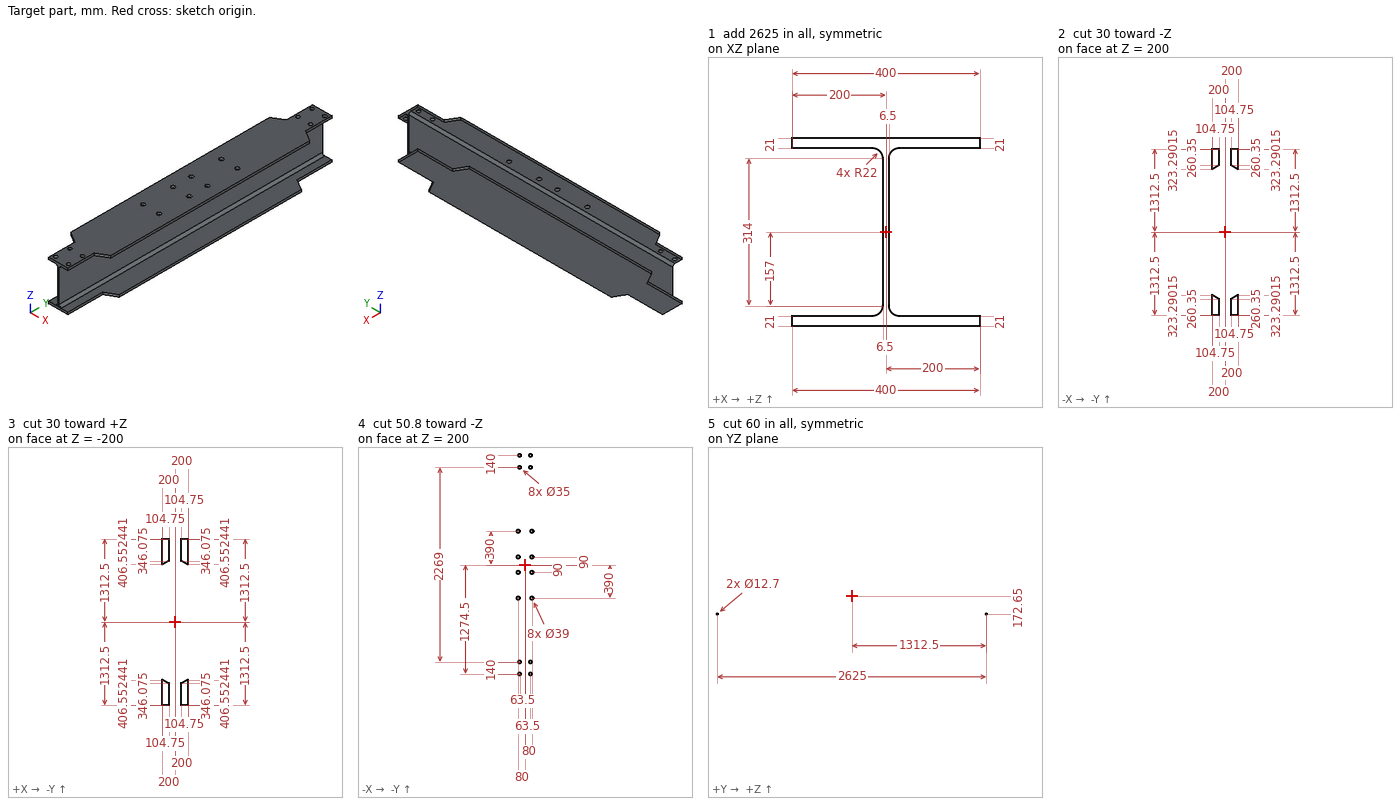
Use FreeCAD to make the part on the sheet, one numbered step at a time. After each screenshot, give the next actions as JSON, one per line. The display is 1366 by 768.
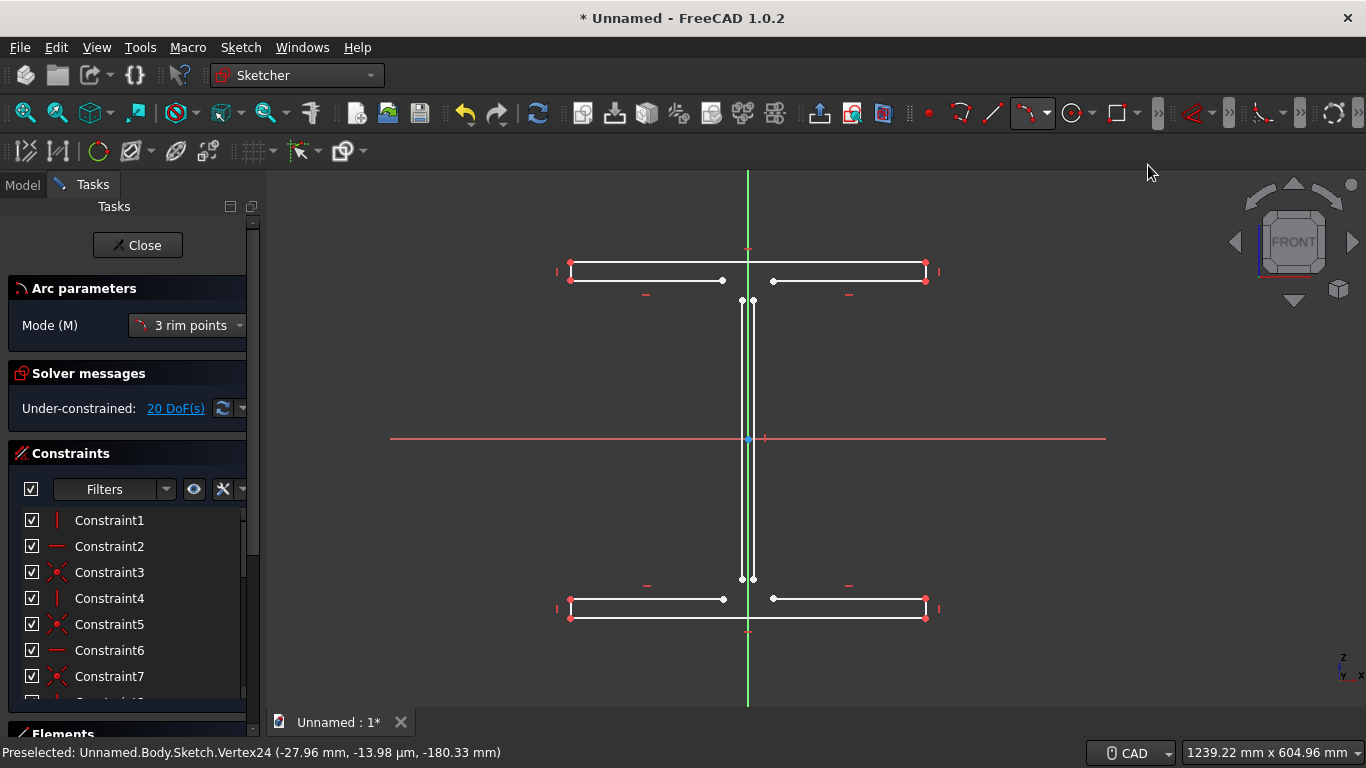
{"action": "scroll", "coordinate": [742, 300], "scroll_direction": "up", "scroll_amount": 6}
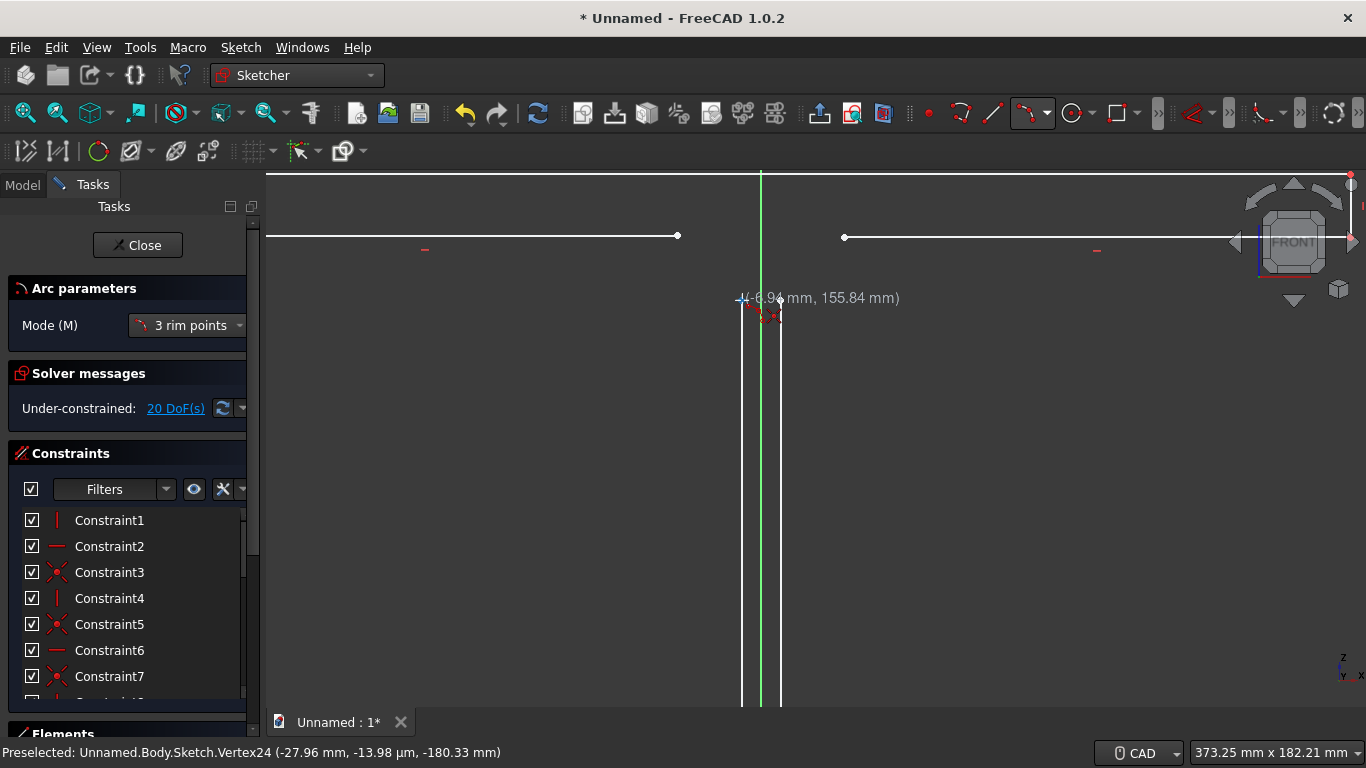
{"action": "left_click", "coordinate": [742, 300]}
{"action": "left_click", "coordinate": [677, 236]}
{"action": "left_click", "coordinate": [723, 253]}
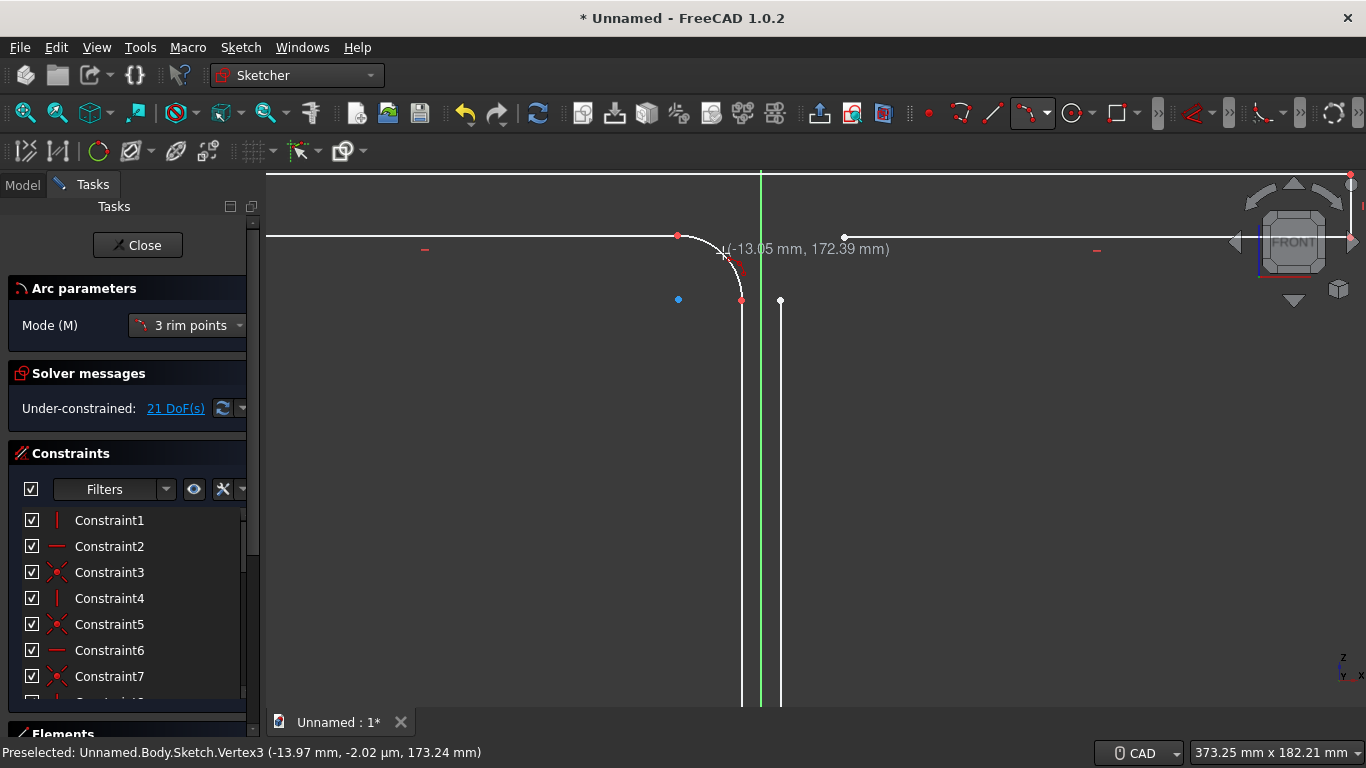
{"action": "left_click", "coordinate": [844, 237]}
{"action": "left_click", "coordinate": [781, 301]}
{"action": "left_click", "coordinate": [800, 253]}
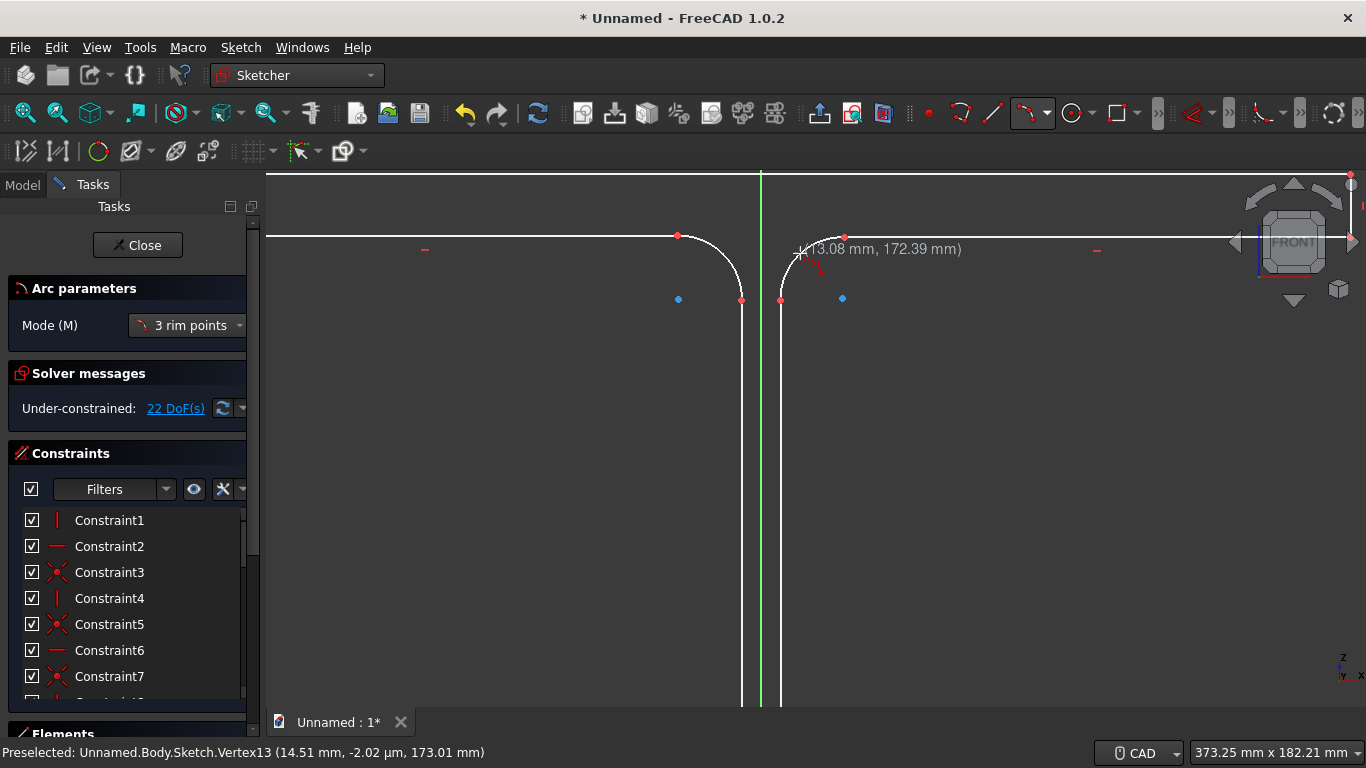
{"action": "scroll", "coordinate": [741, 299], "scroll_direction": "down", "scroll_amount": 6}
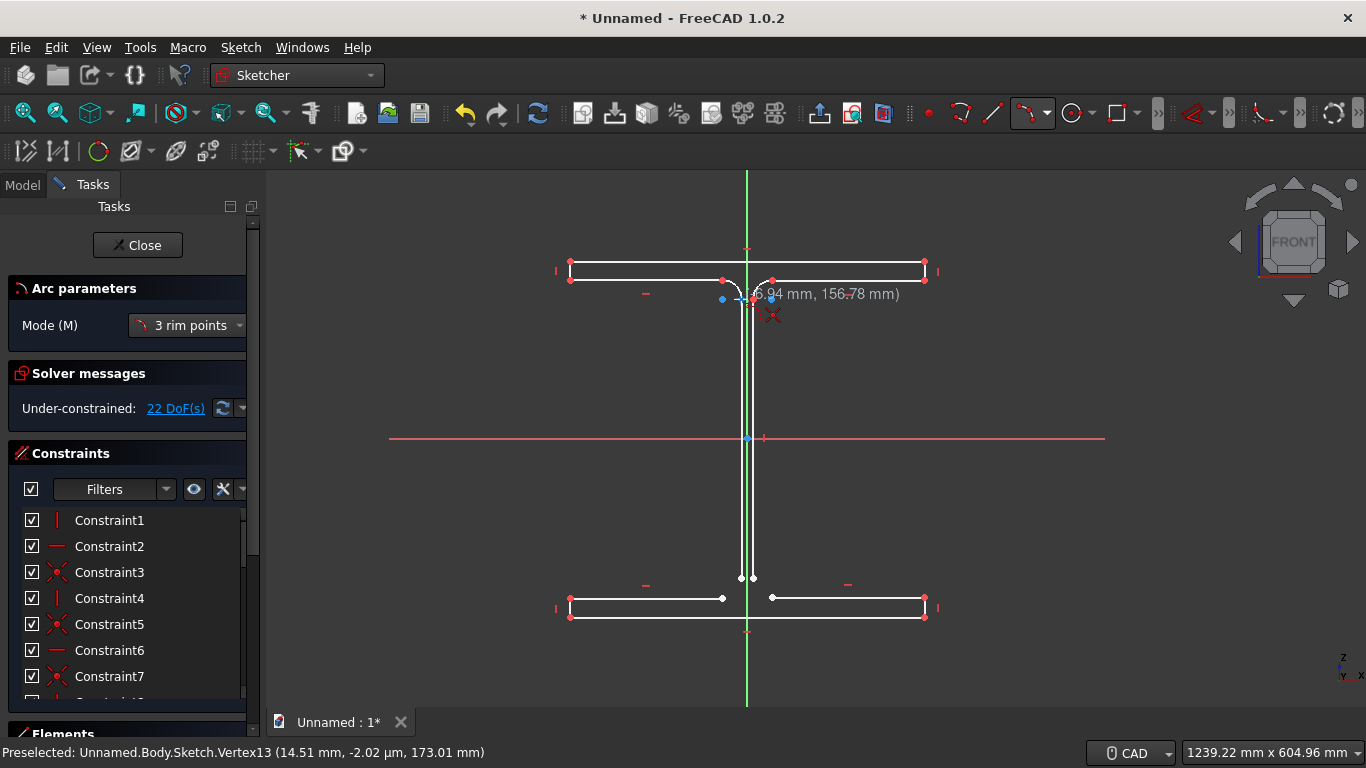
{"action": "scroll", "coordinate": [753, 578], "scroll_direction": "up", "scroll_amount": 6}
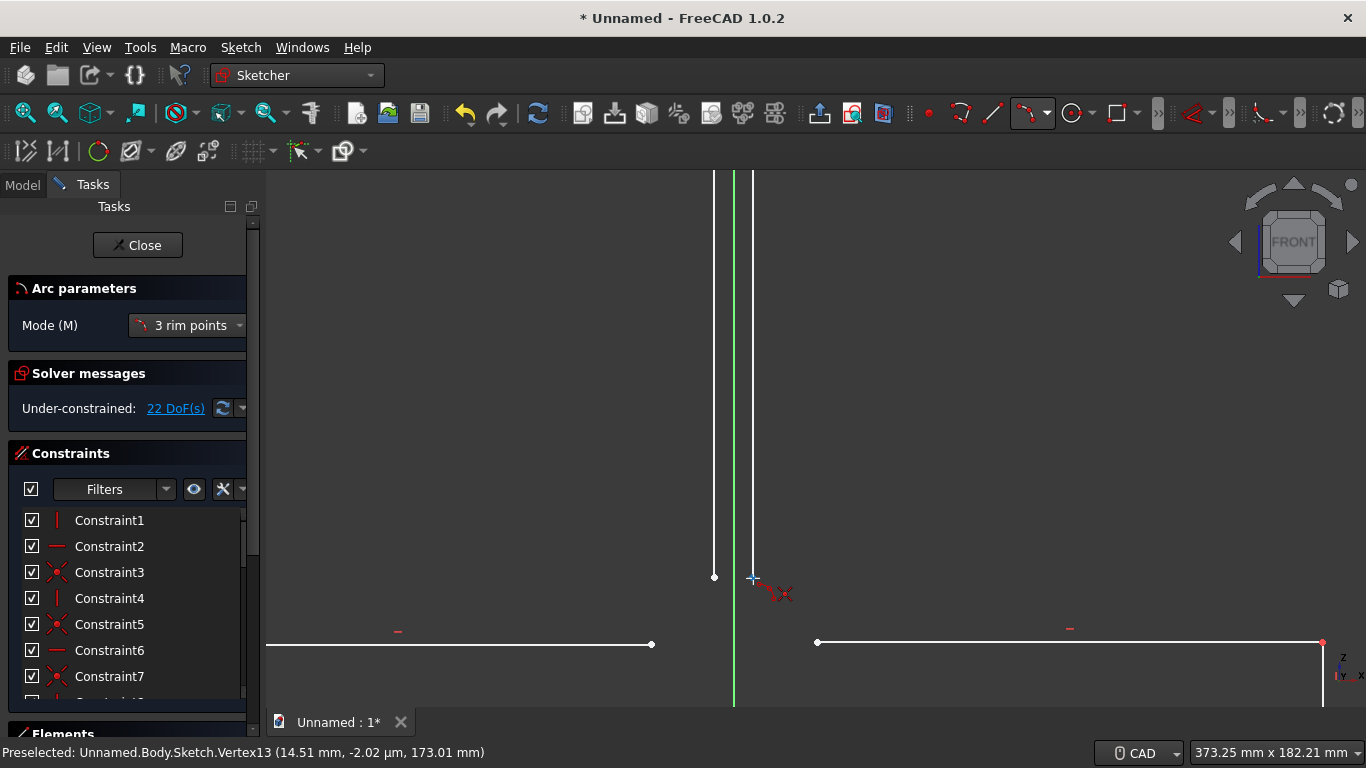
{"action": "left_click", "coordinate": [753, 578]}
{"action": "left_click", "coordinate": [818, 642]}
{"action": "left_click", "coordinate": [772, 622]}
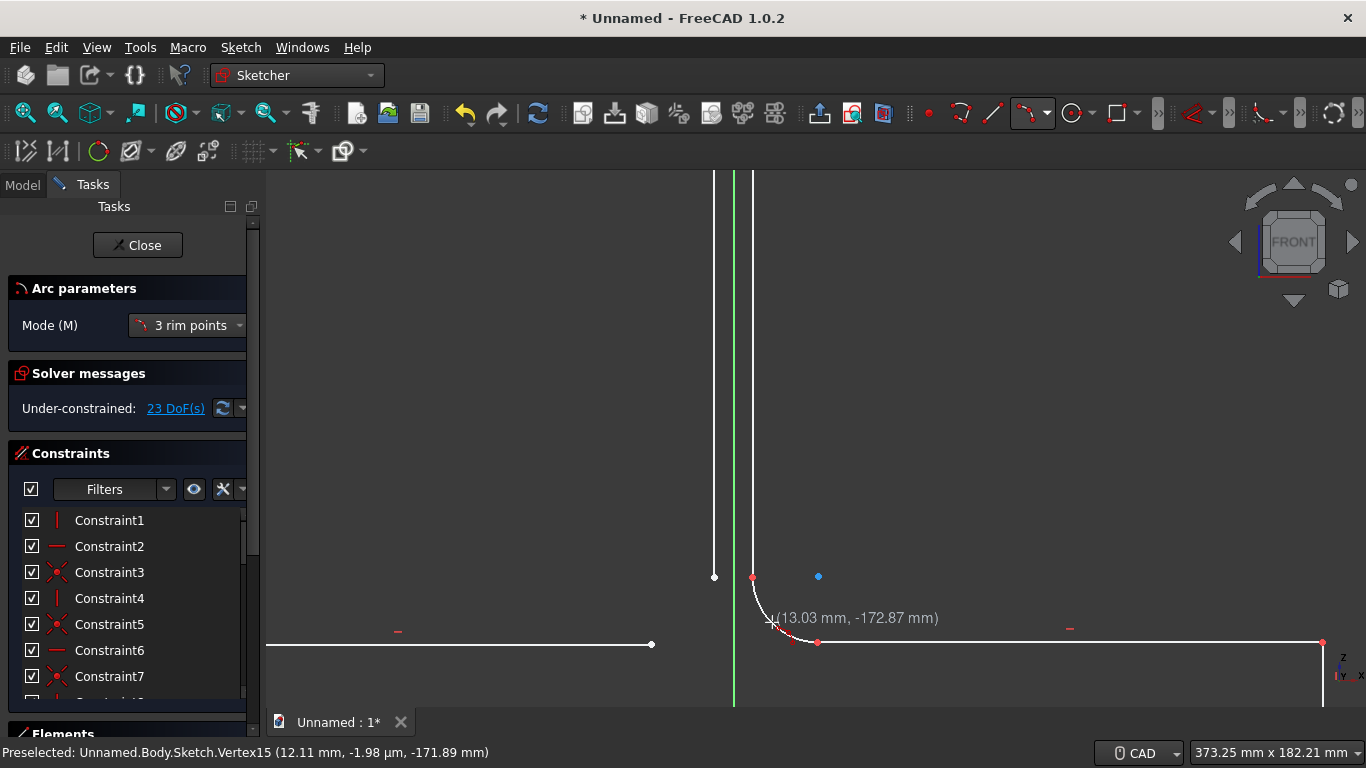
{"action": "left_click", "coordinate": [651, 645]}
{"action": "left_click", "coordinate": [714, 577]}
{"action": "left_click", "coordinate": [695, 622]}
{"action": "key", "text": "Escape"}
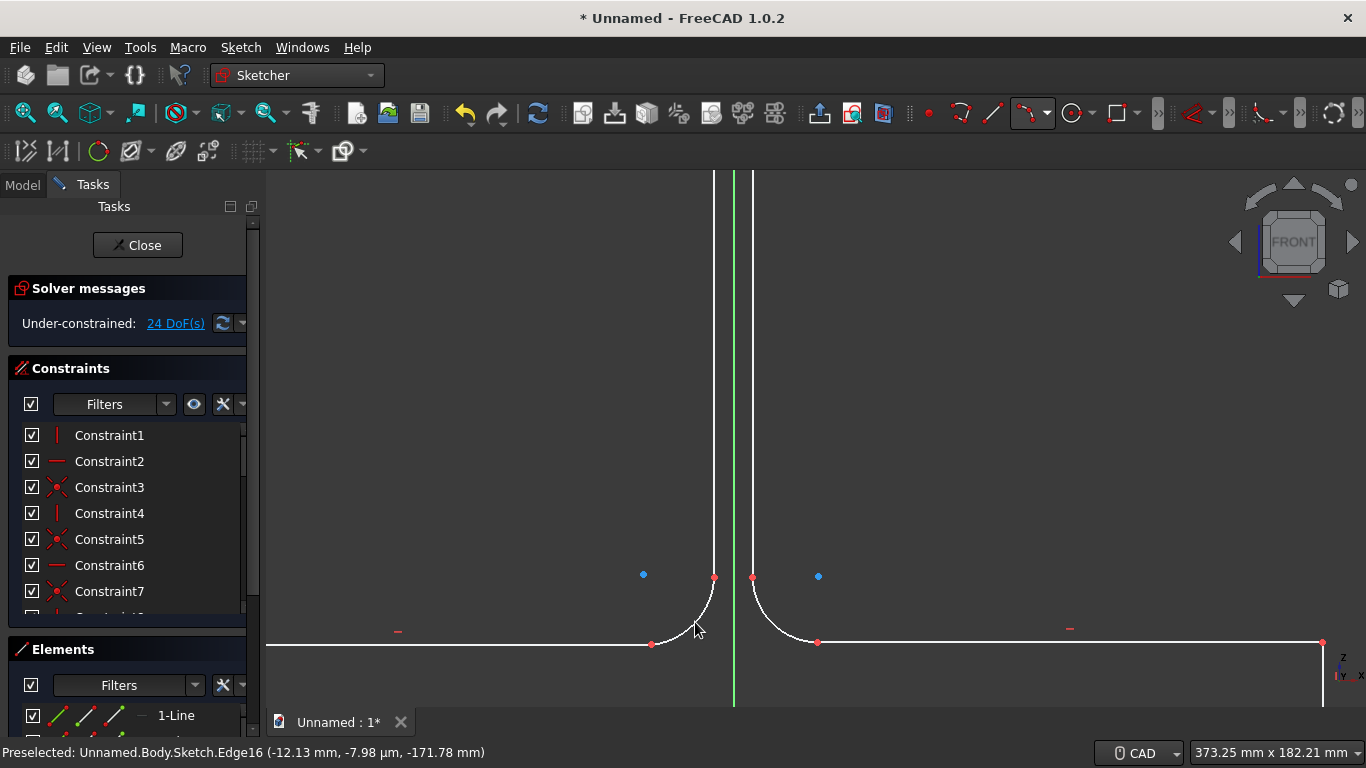
{"action": "left_click", "coordinate": [714, 300]}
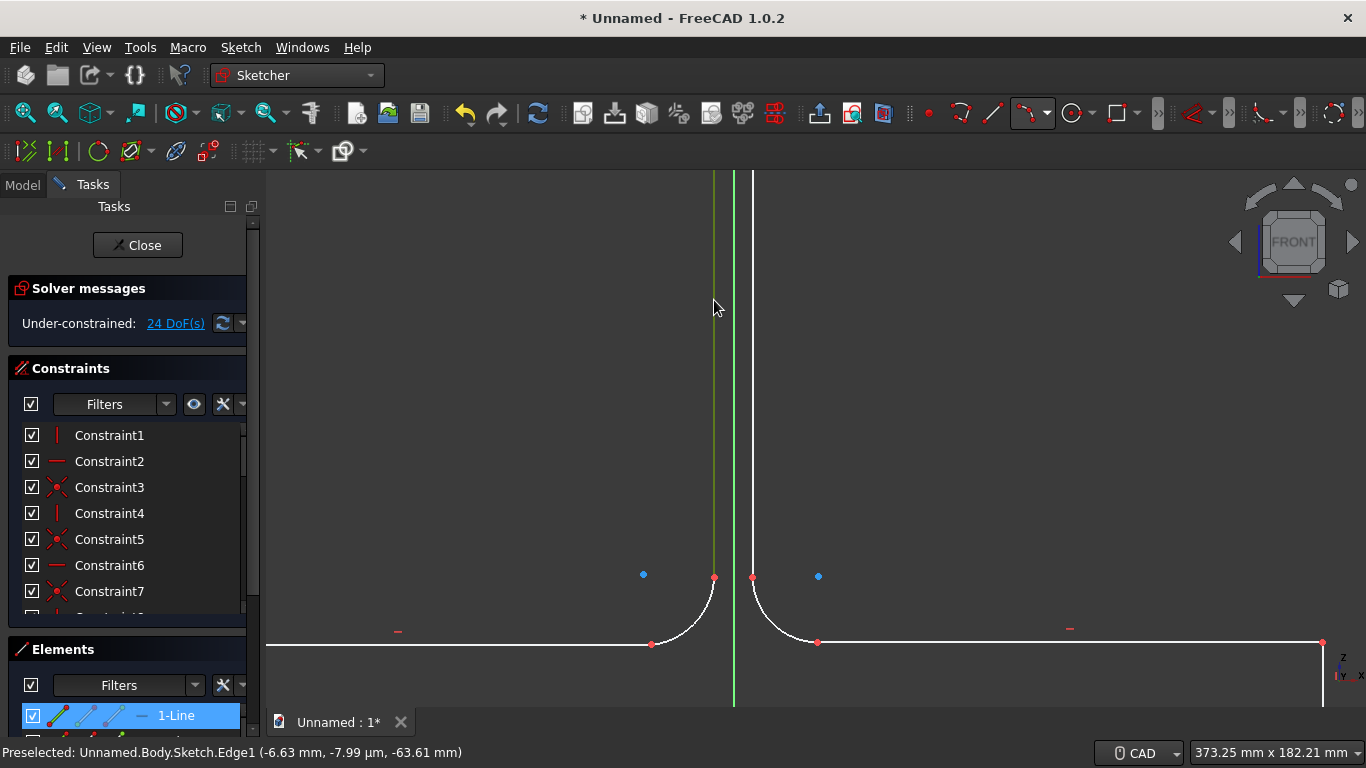
{"action": "scroll", "coordinate": [753, 579], "scroll_direction": "down", "scroll_amount": 6}